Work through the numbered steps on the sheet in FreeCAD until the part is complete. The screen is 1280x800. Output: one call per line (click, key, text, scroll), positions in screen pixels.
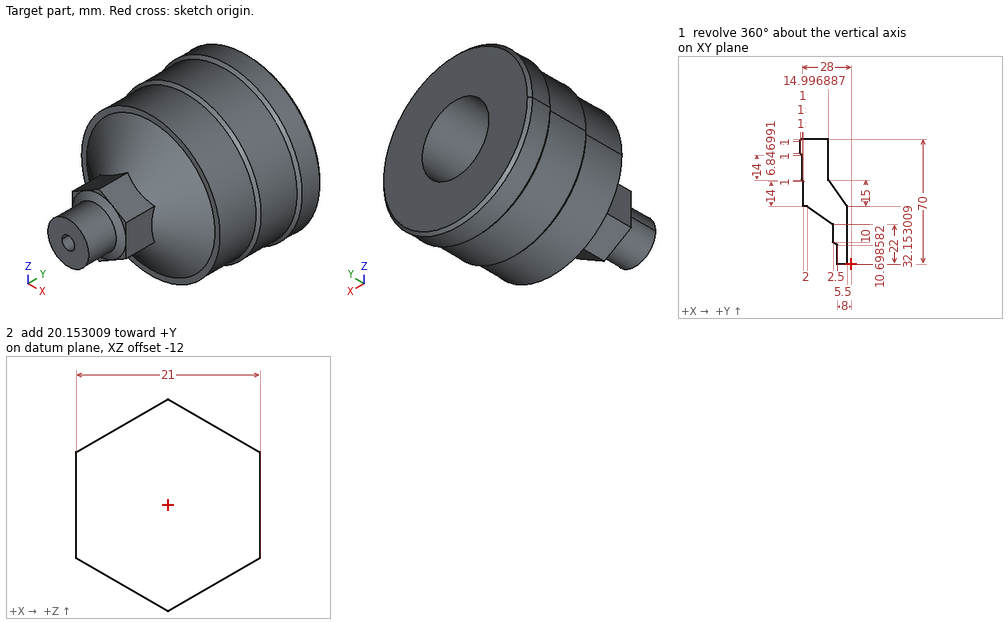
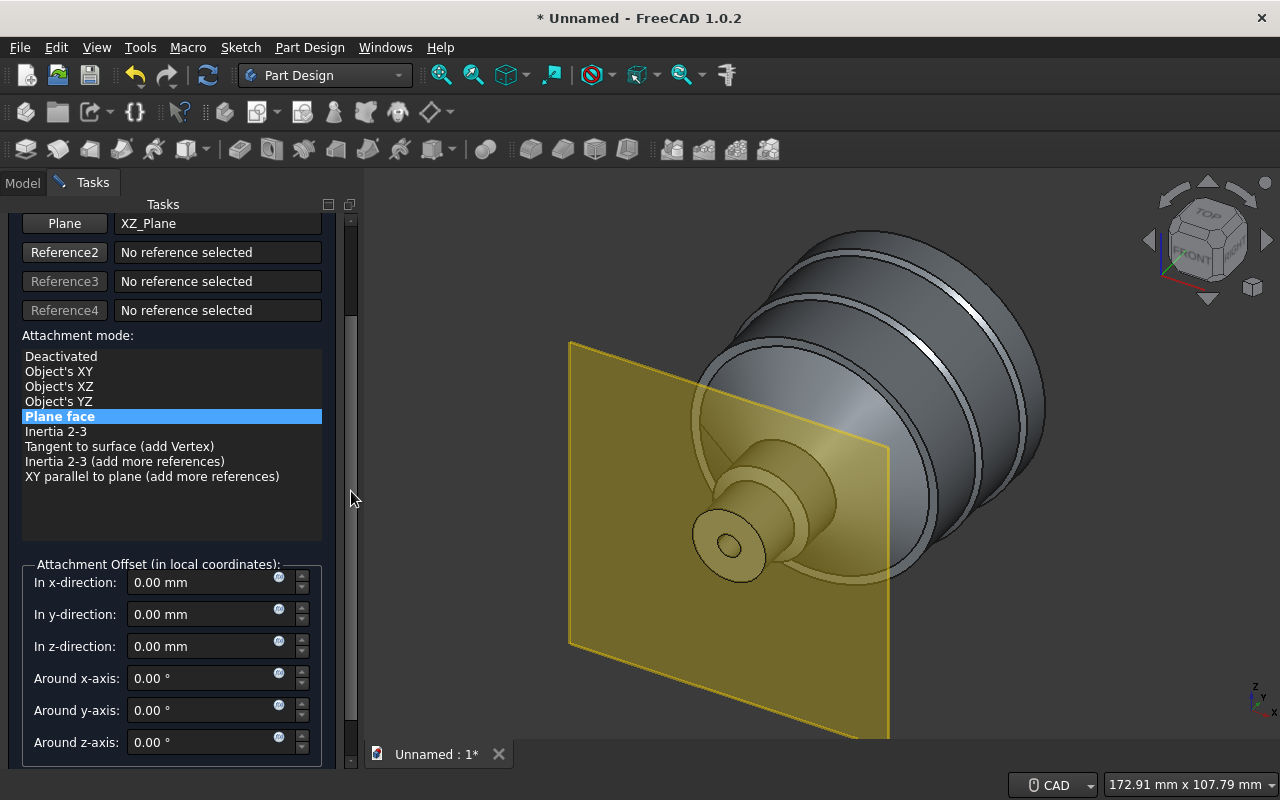
triple_click(210, 646)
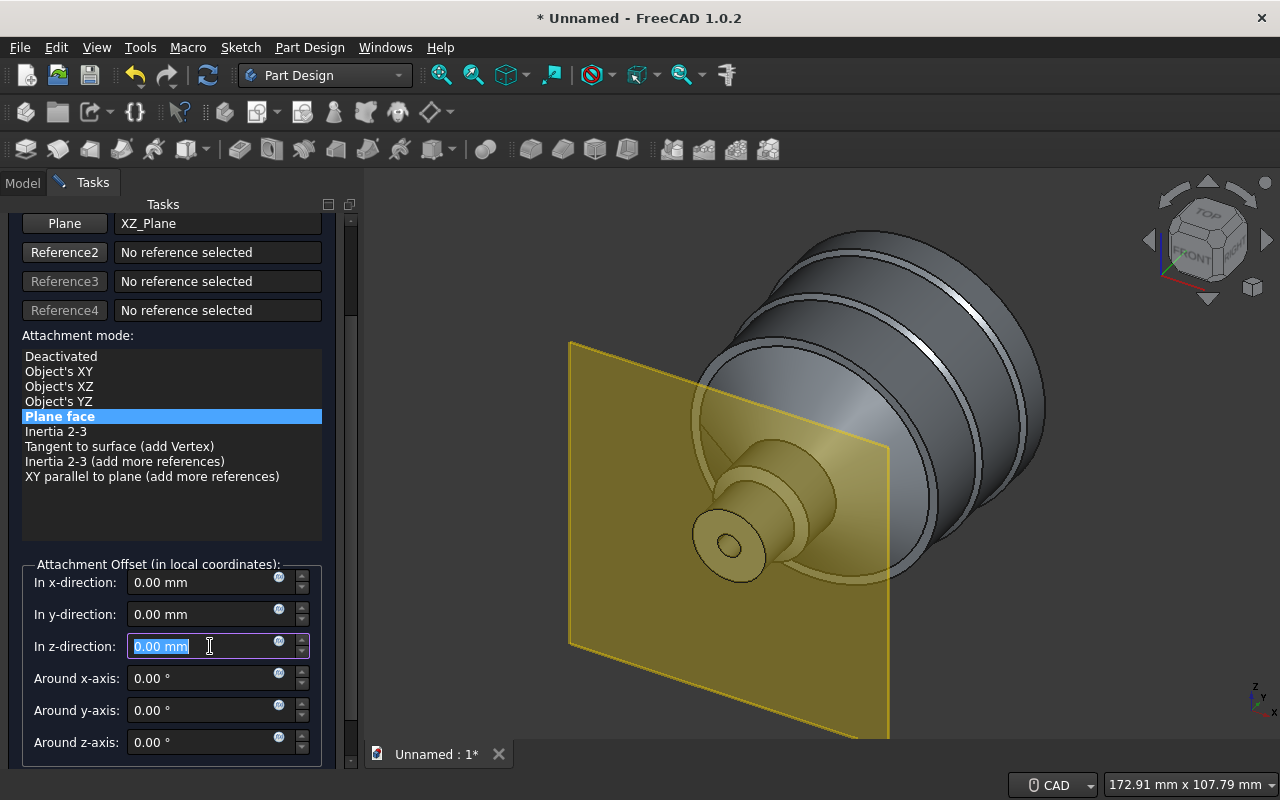
text(-12)
key(Tab)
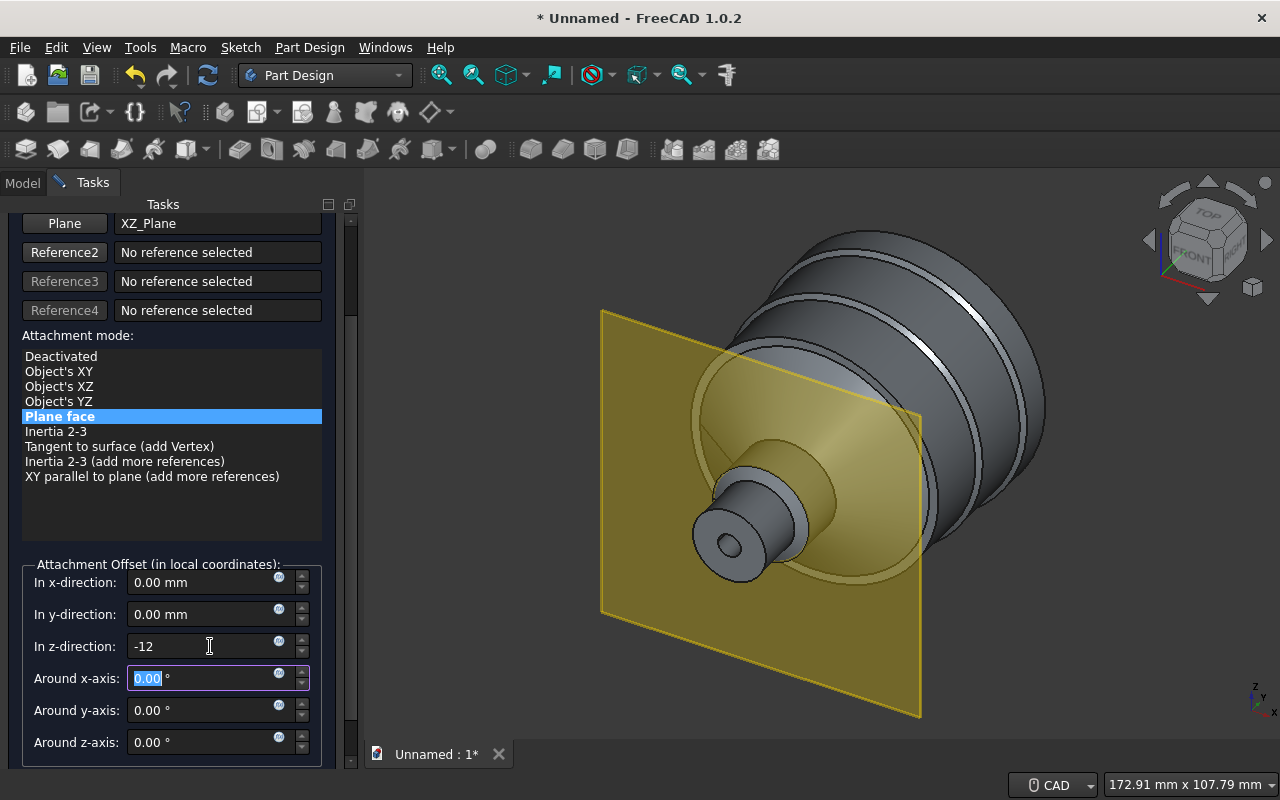
scroll(351, 491, up, 3)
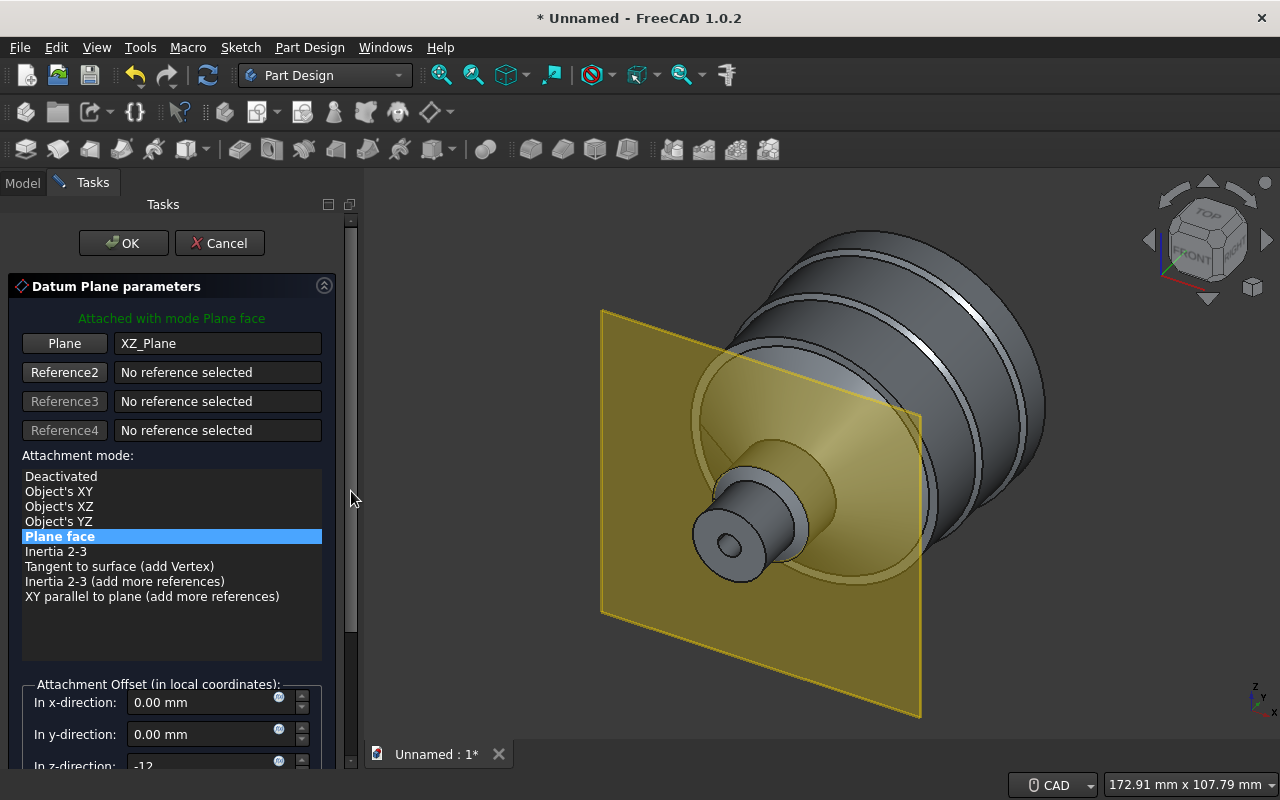
click(124, 243)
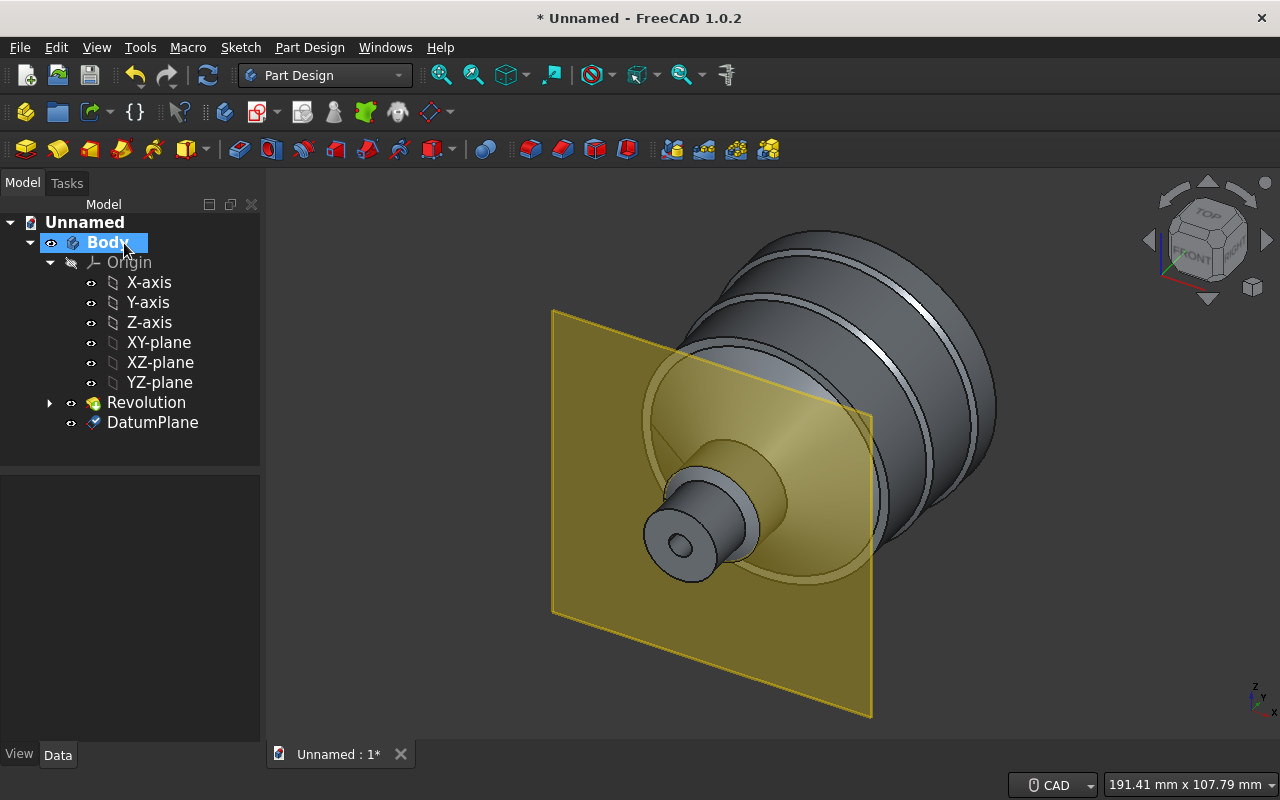
click(116, 423)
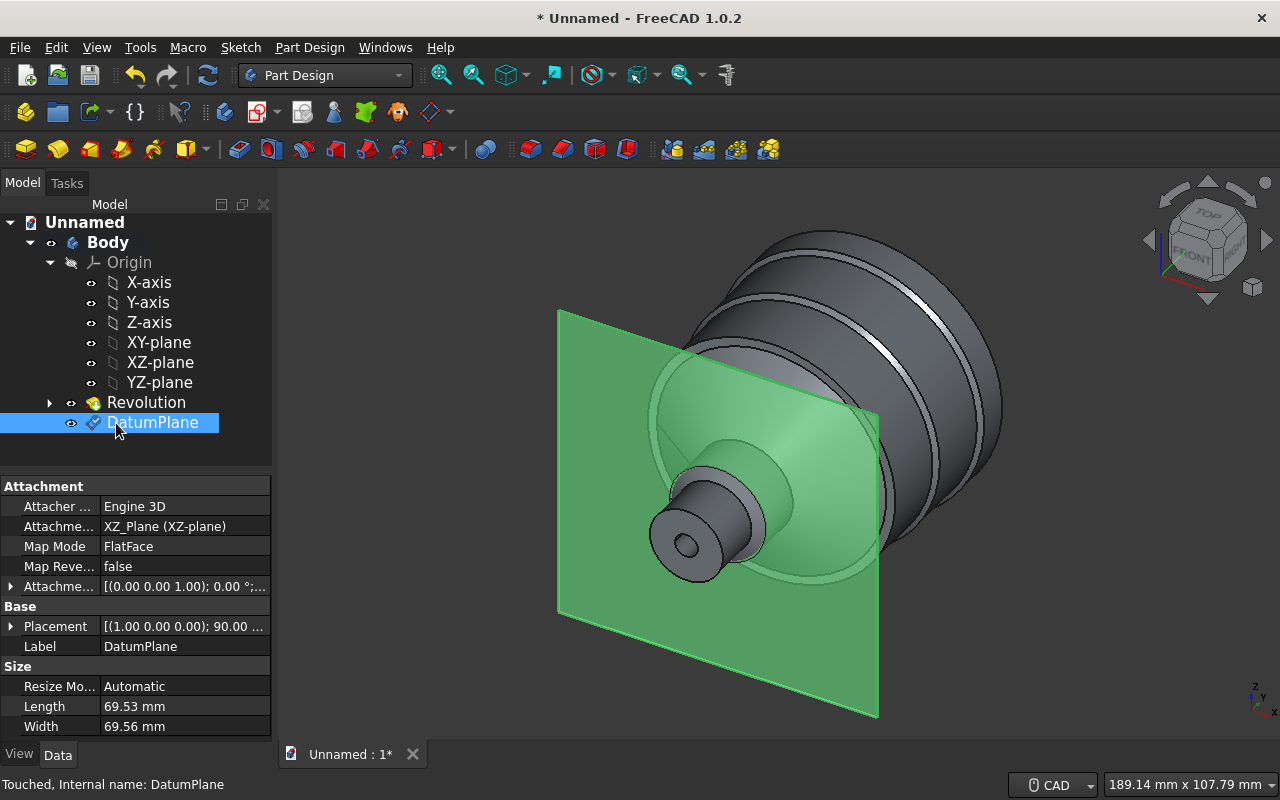
click(258, 112)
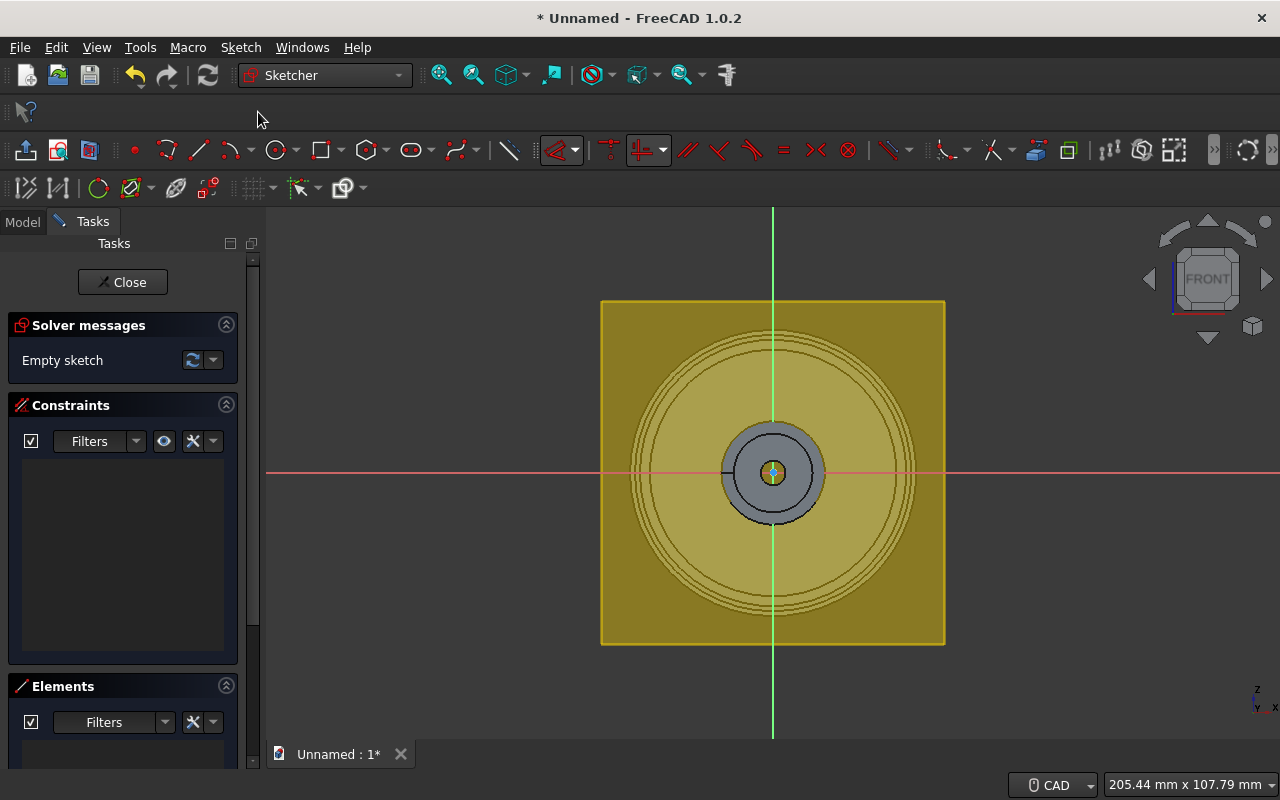
click(90, 150)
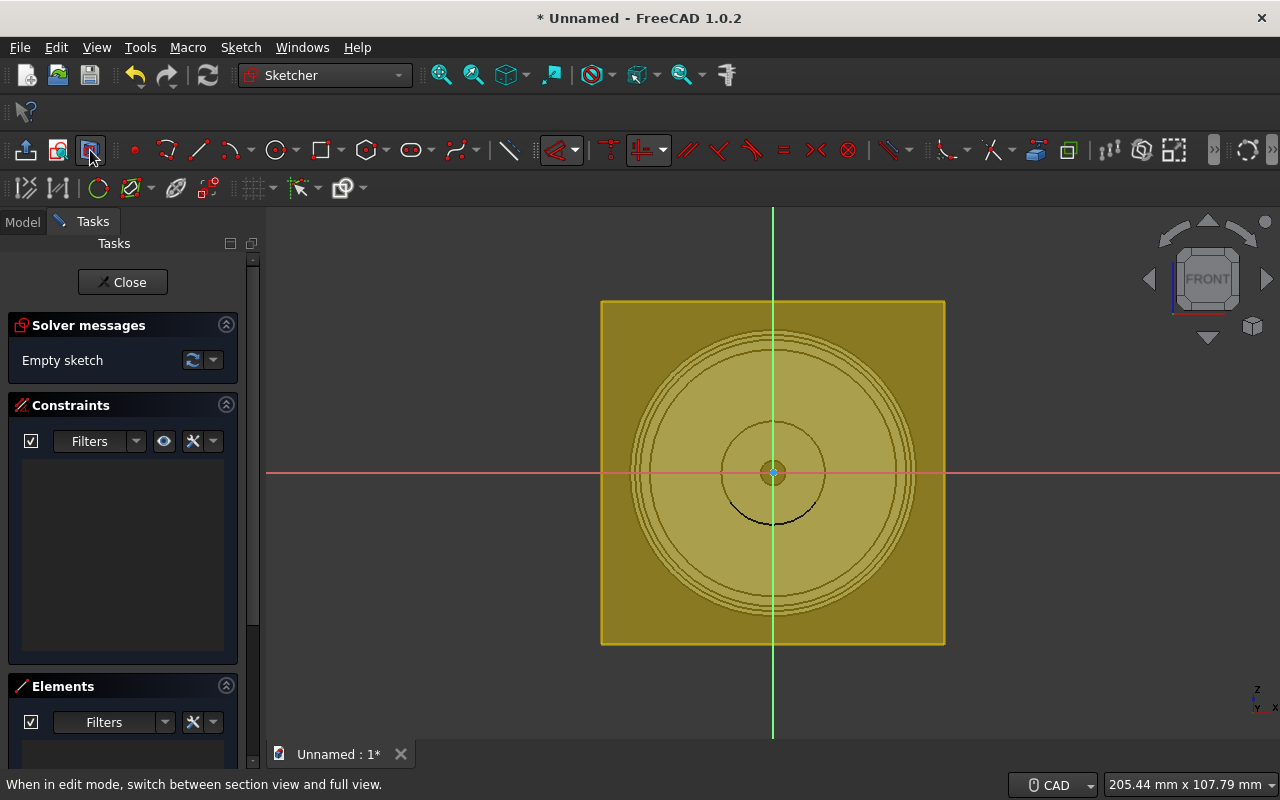
scroll(813, 473, up, 5)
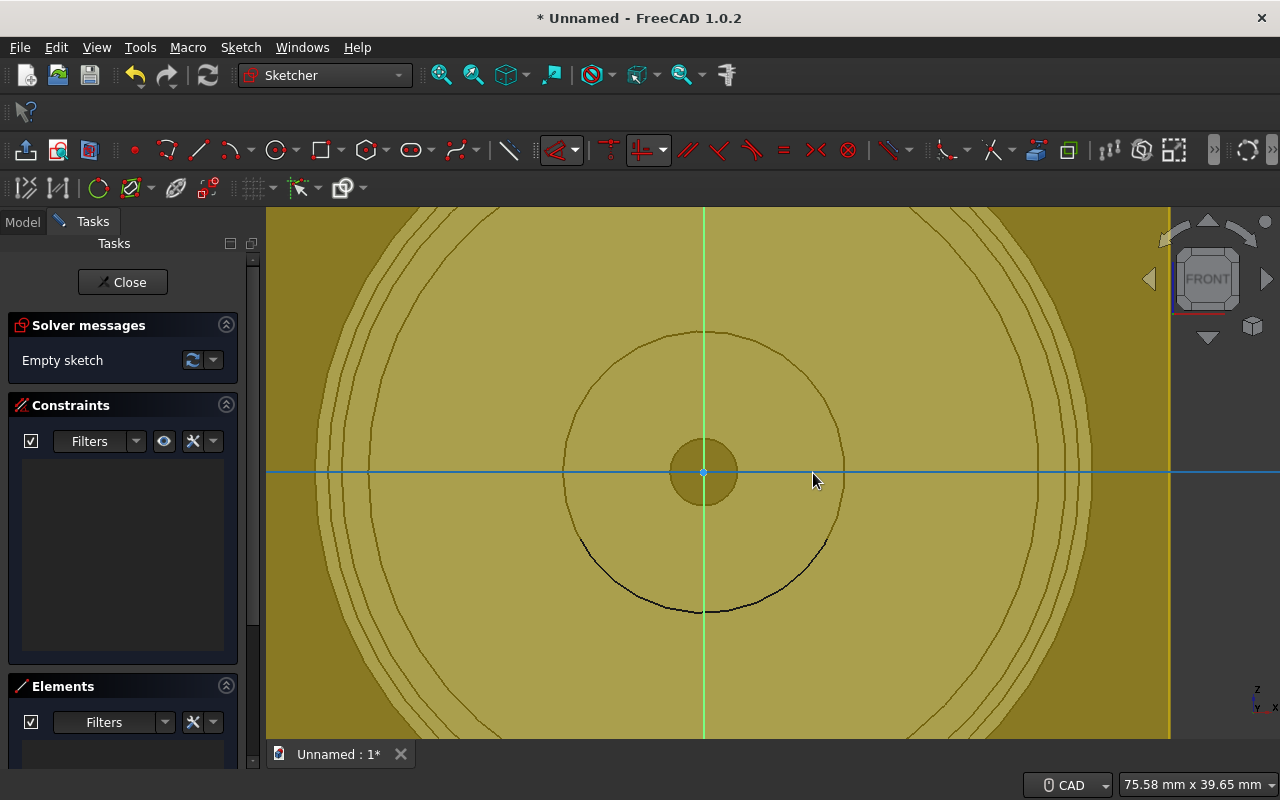
click(366, 150)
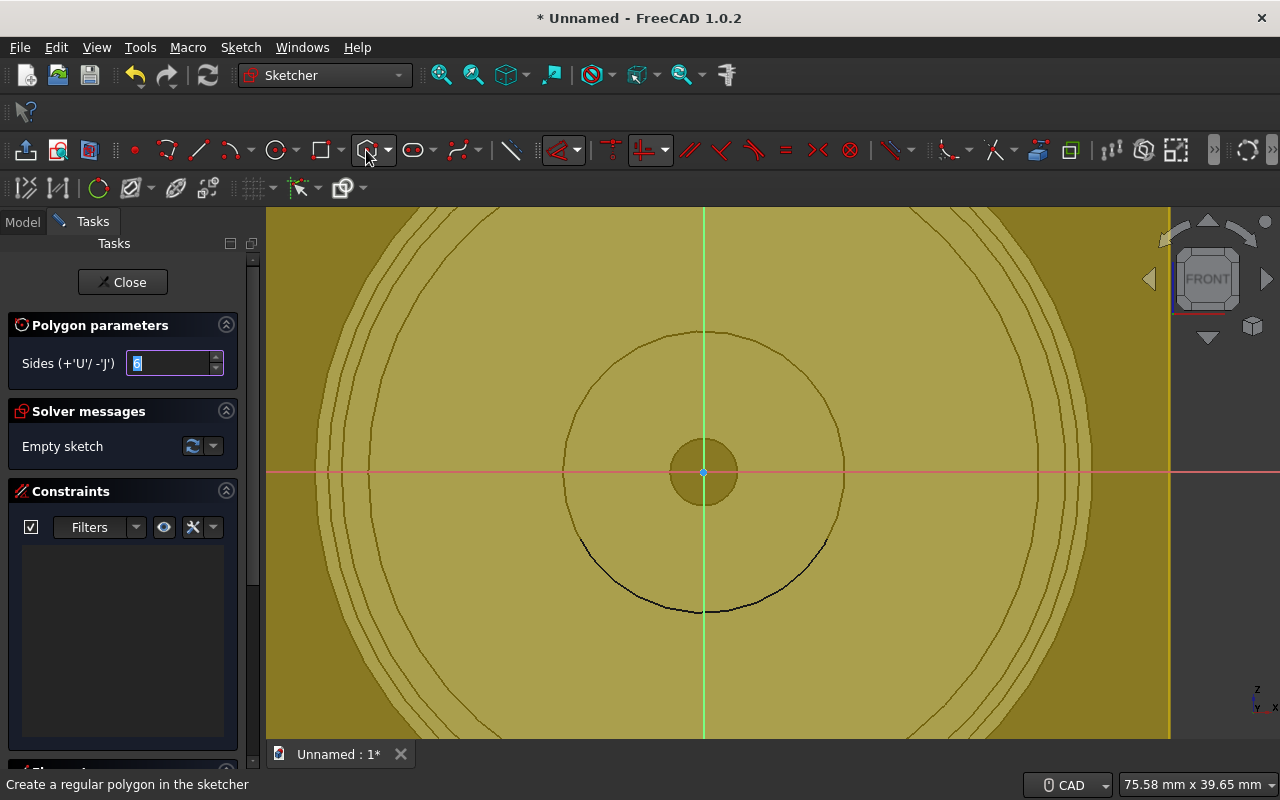
click(704, 472)